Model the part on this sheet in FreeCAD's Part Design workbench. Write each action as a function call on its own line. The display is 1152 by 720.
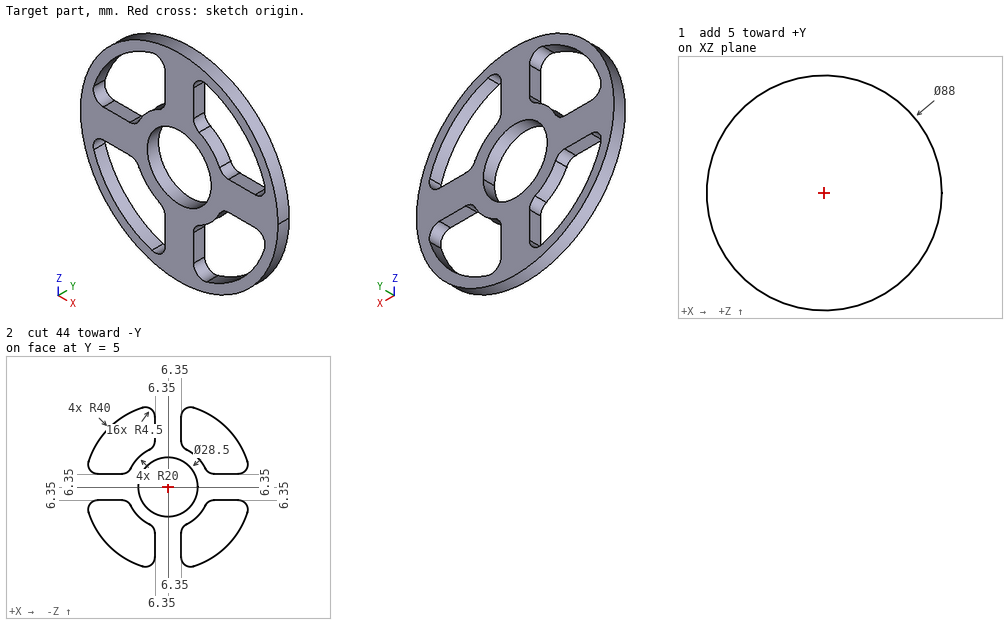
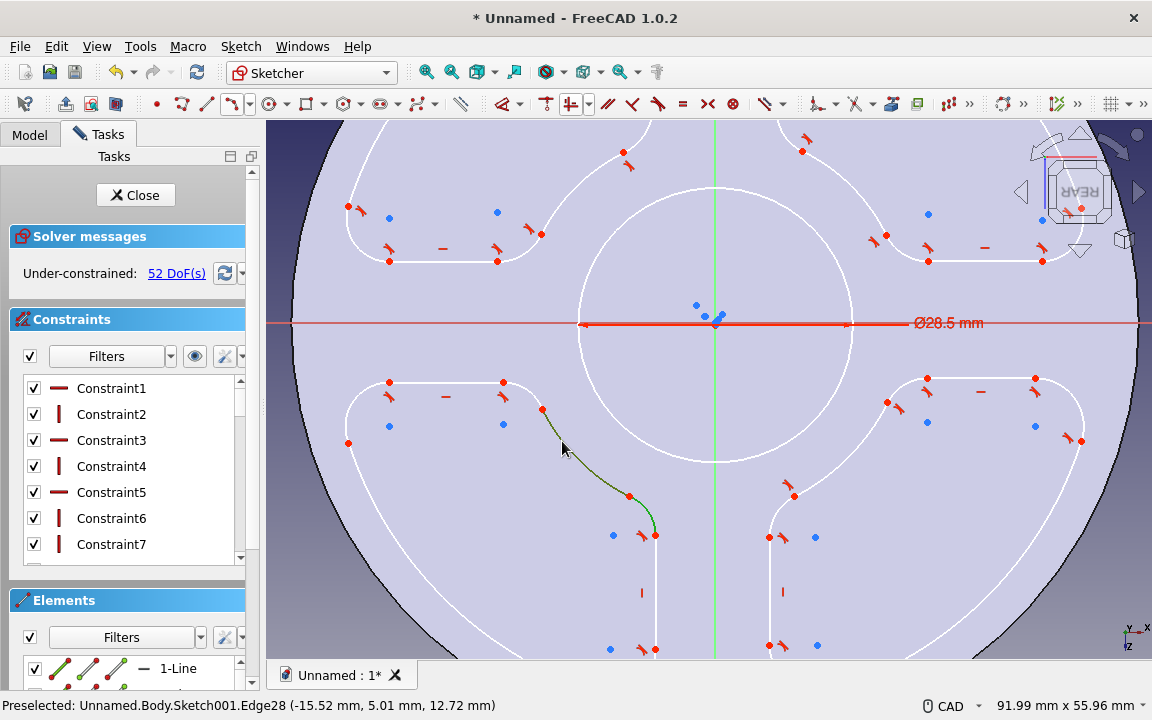
key(t)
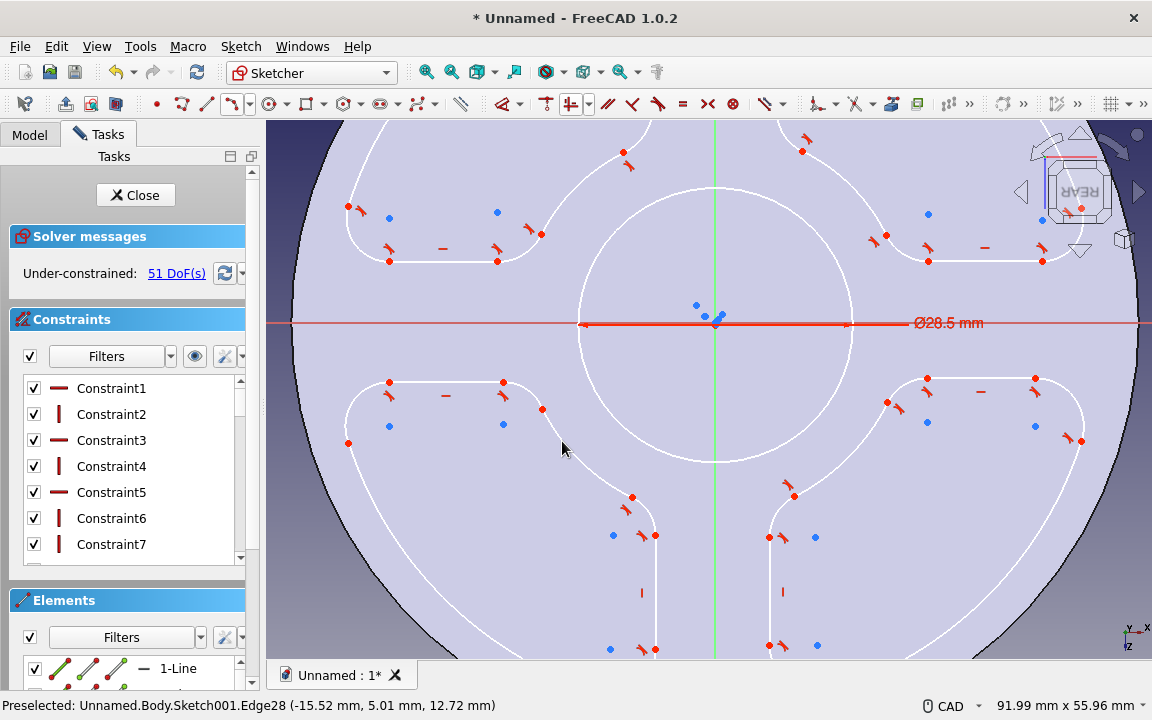
click(563, 442)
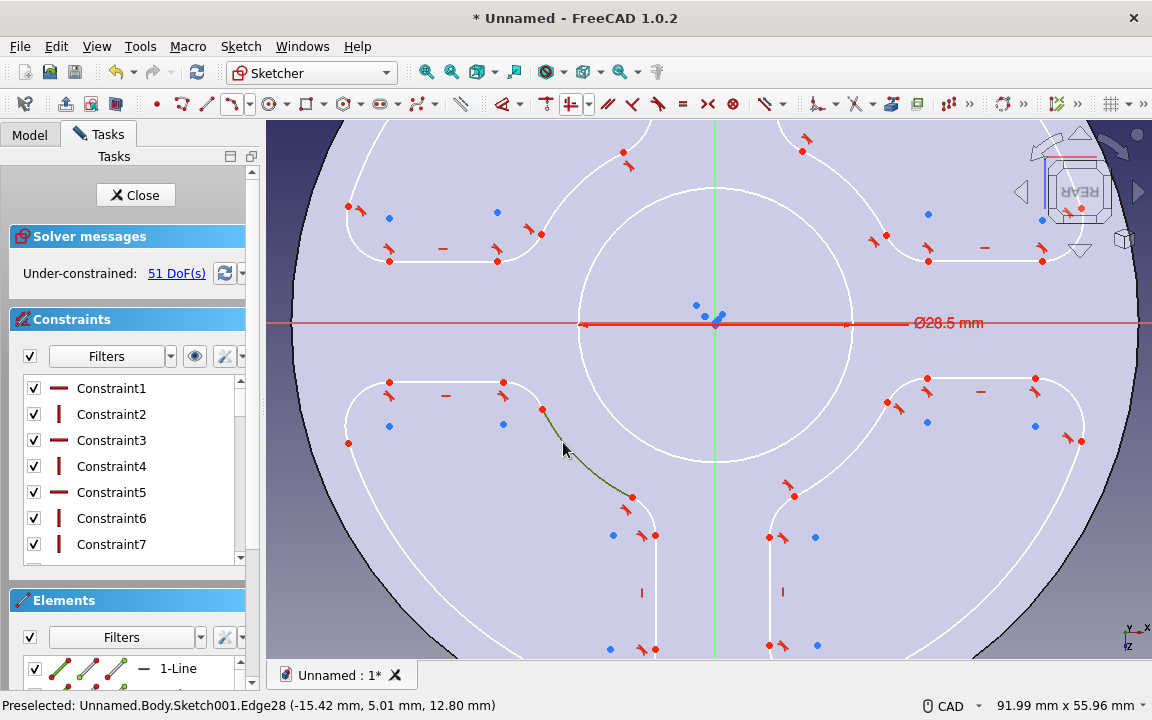
click(535, 397)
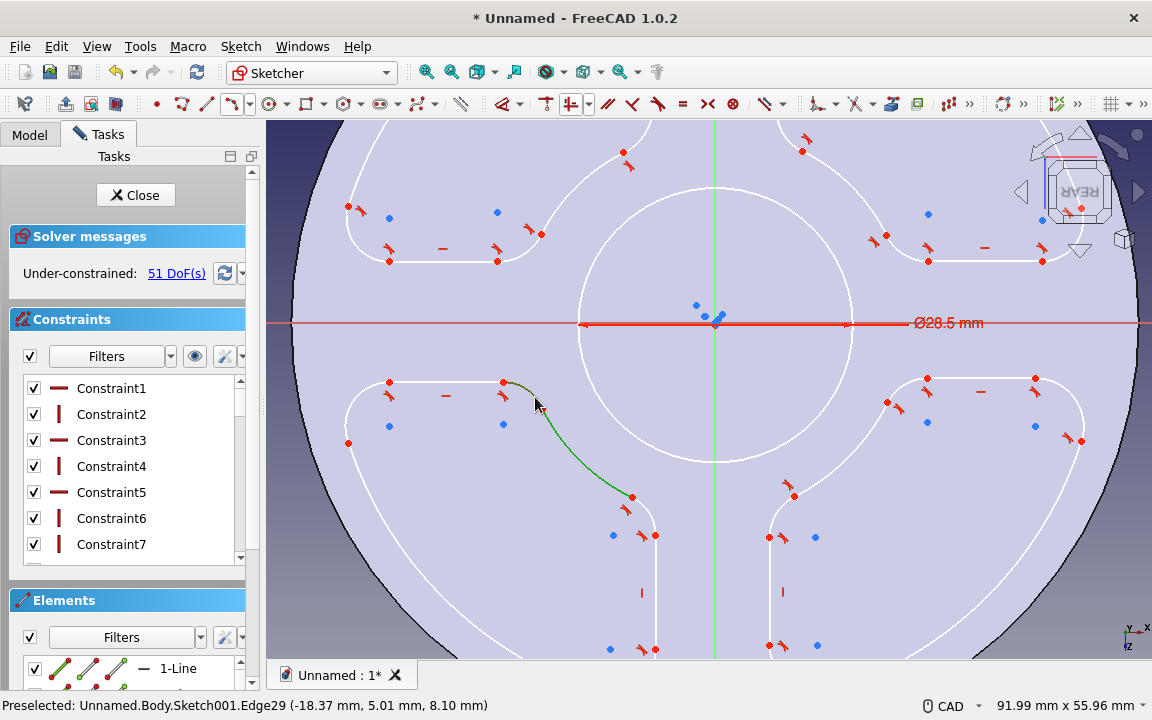
key(t)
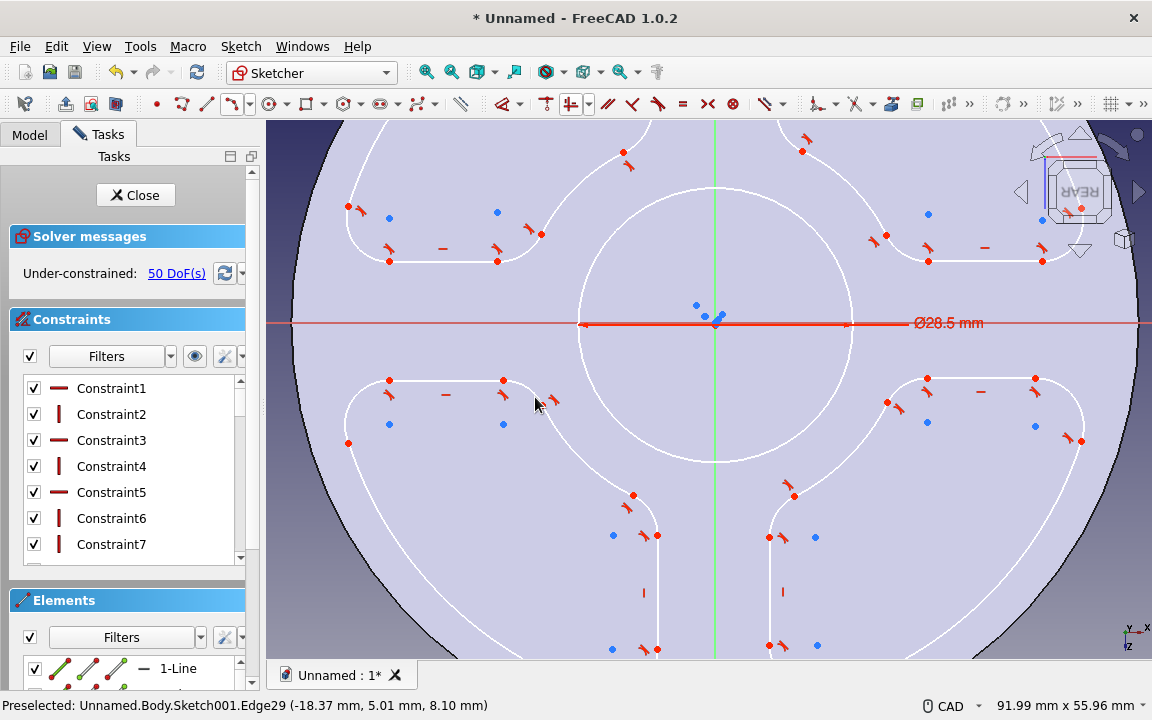
click(364, 388)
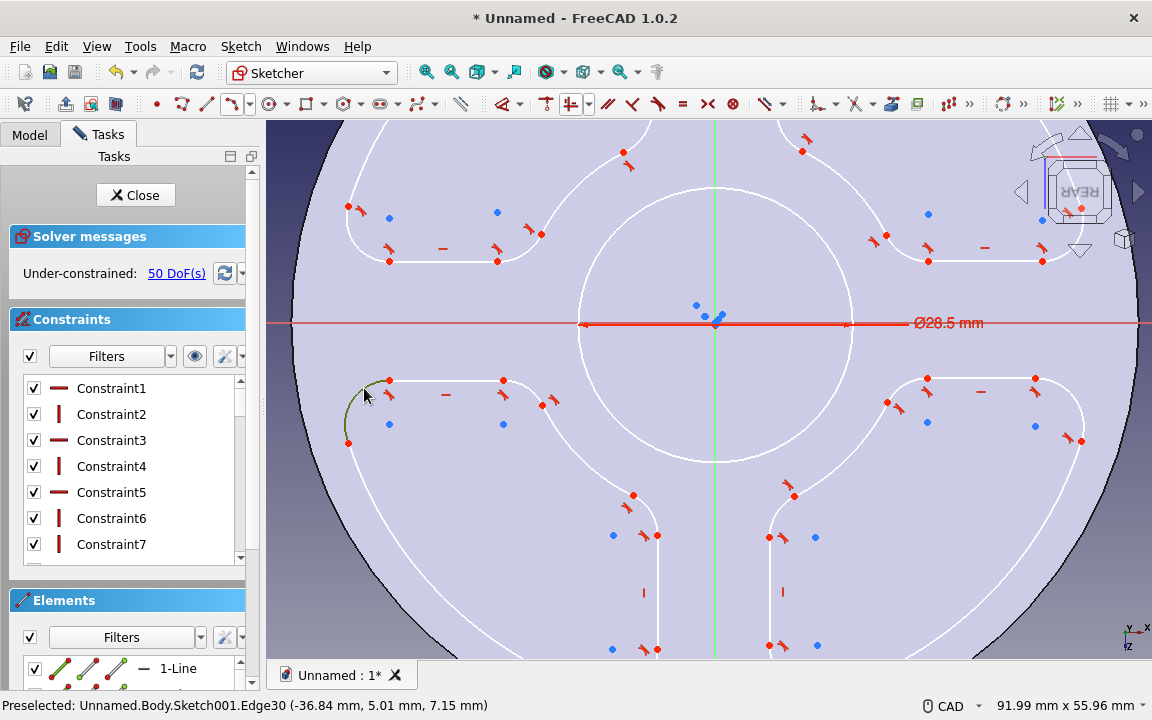
click(397, 541)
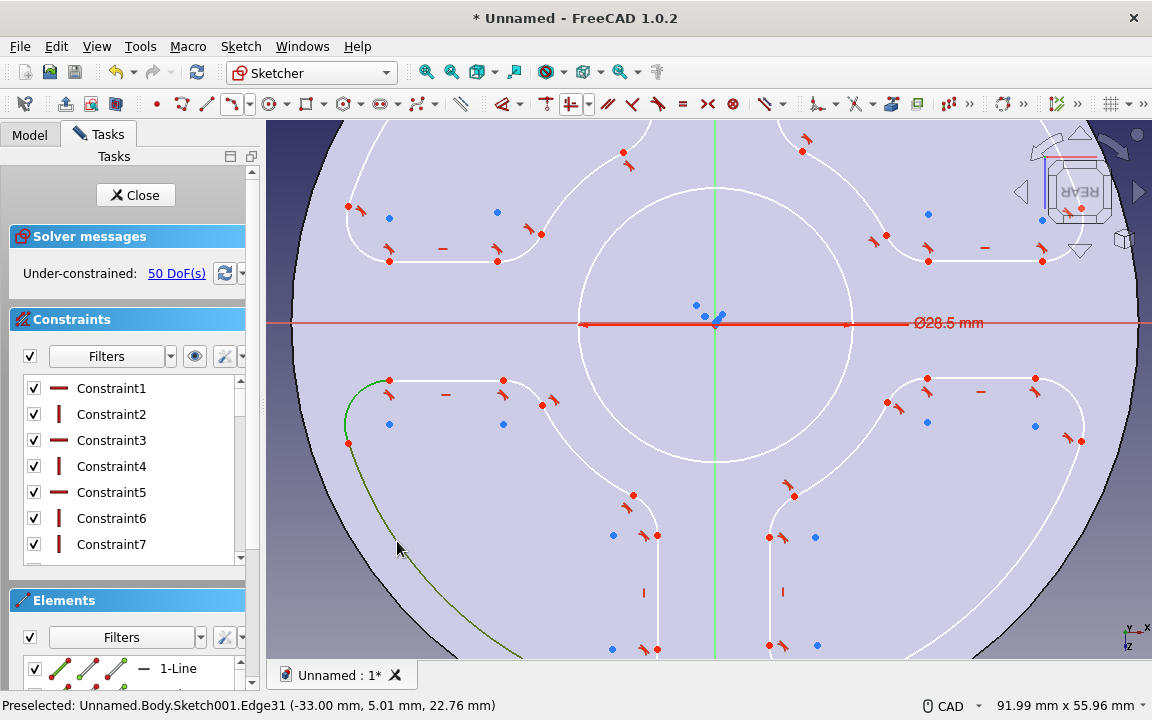
key(t)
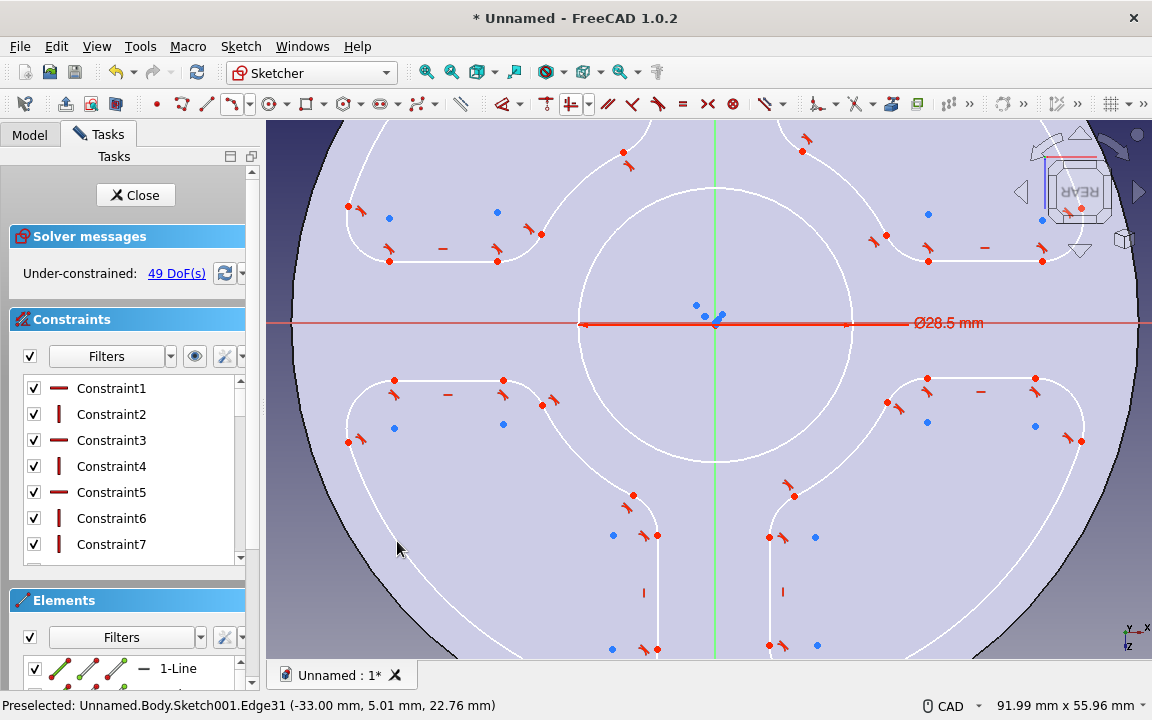
click(397, 541)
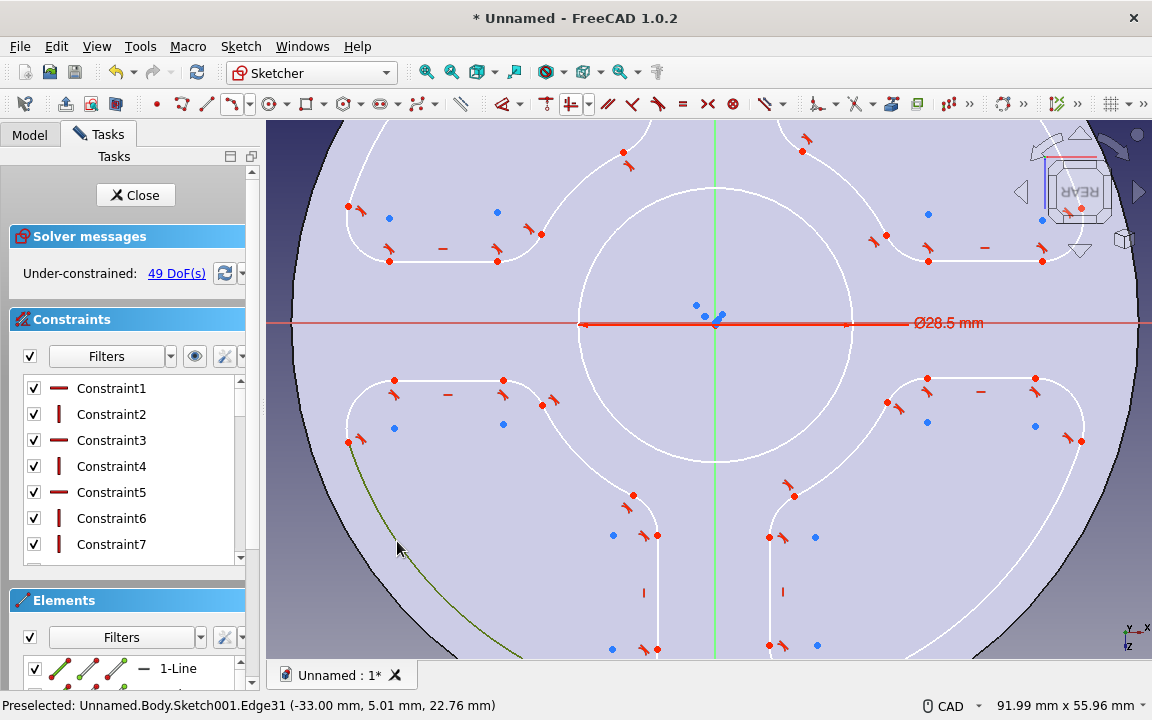
scroll(580, 444, down, 4)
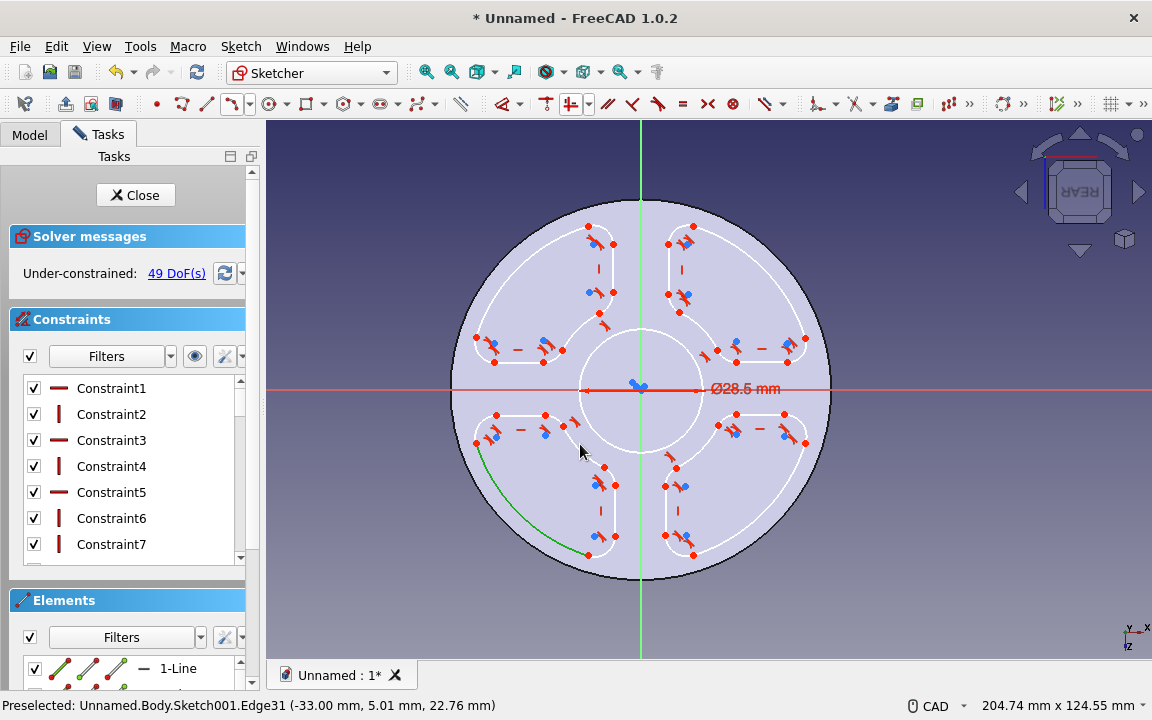
click(600, 556)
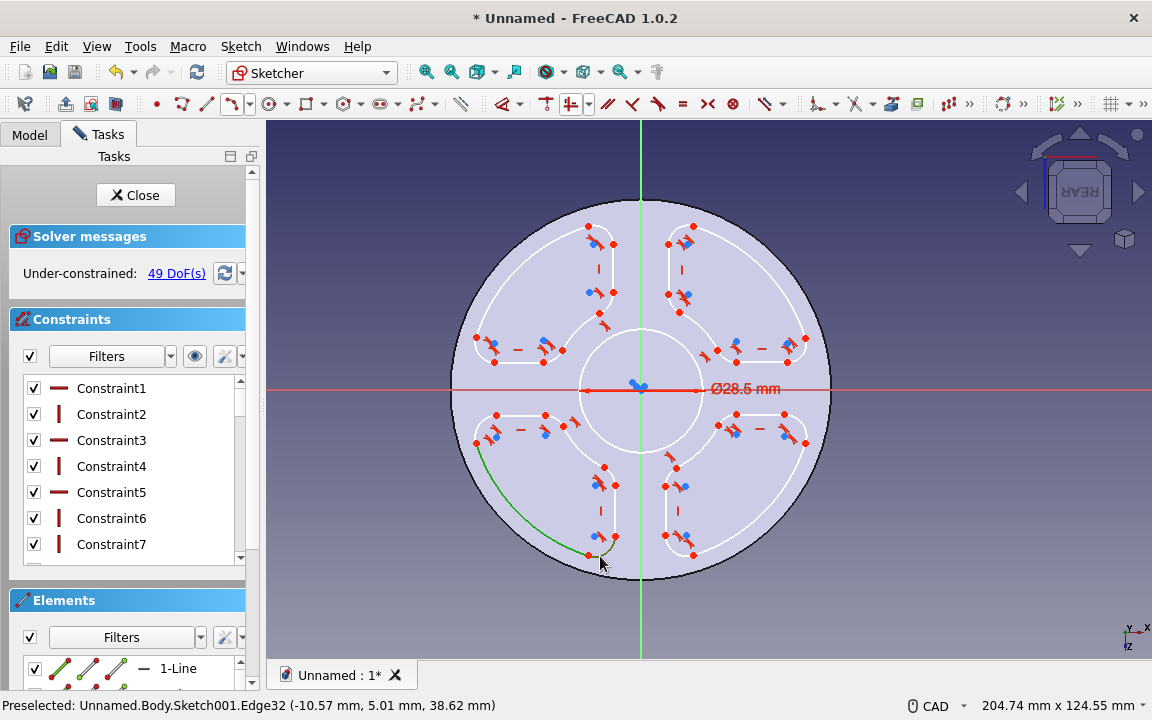
key(t)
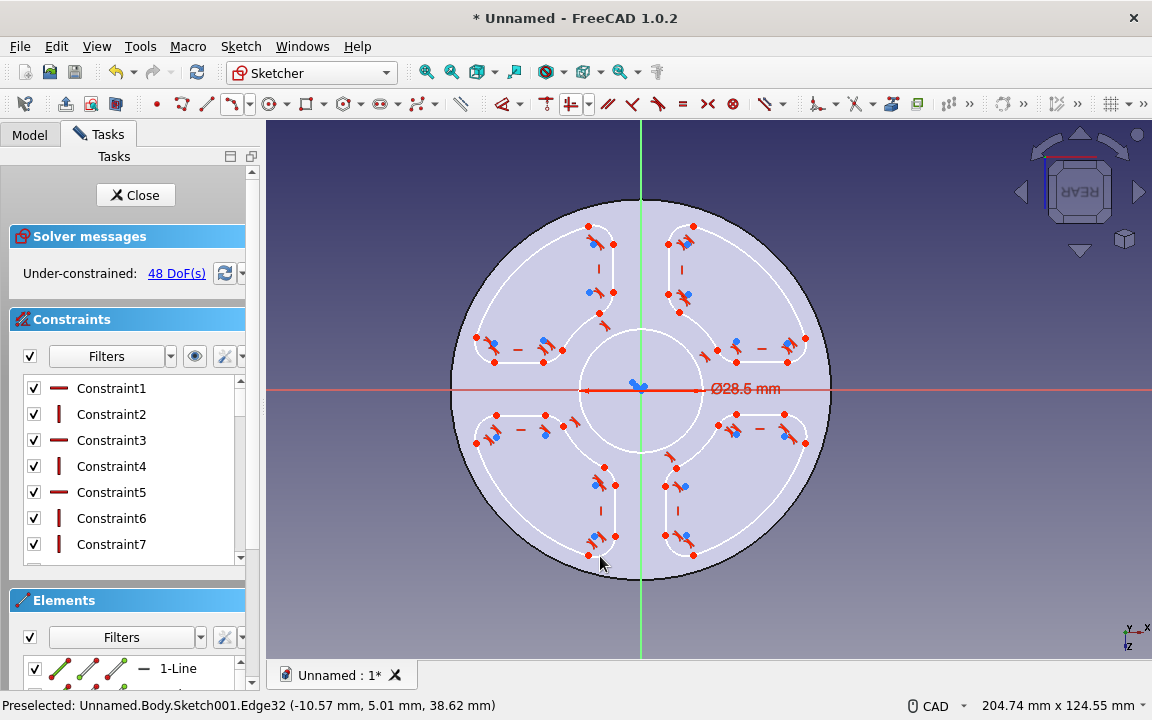
click(685, 347)